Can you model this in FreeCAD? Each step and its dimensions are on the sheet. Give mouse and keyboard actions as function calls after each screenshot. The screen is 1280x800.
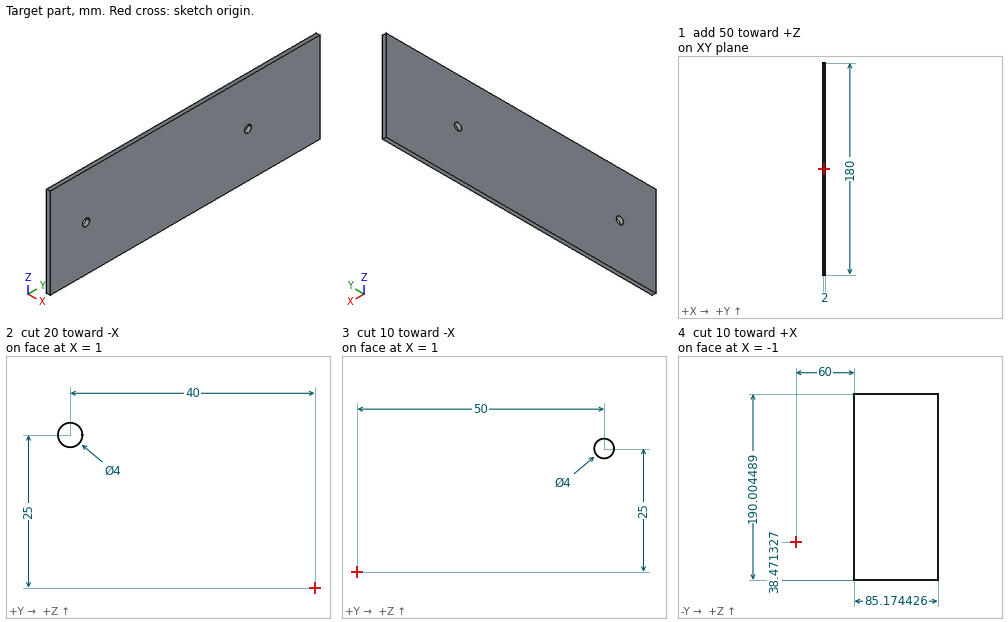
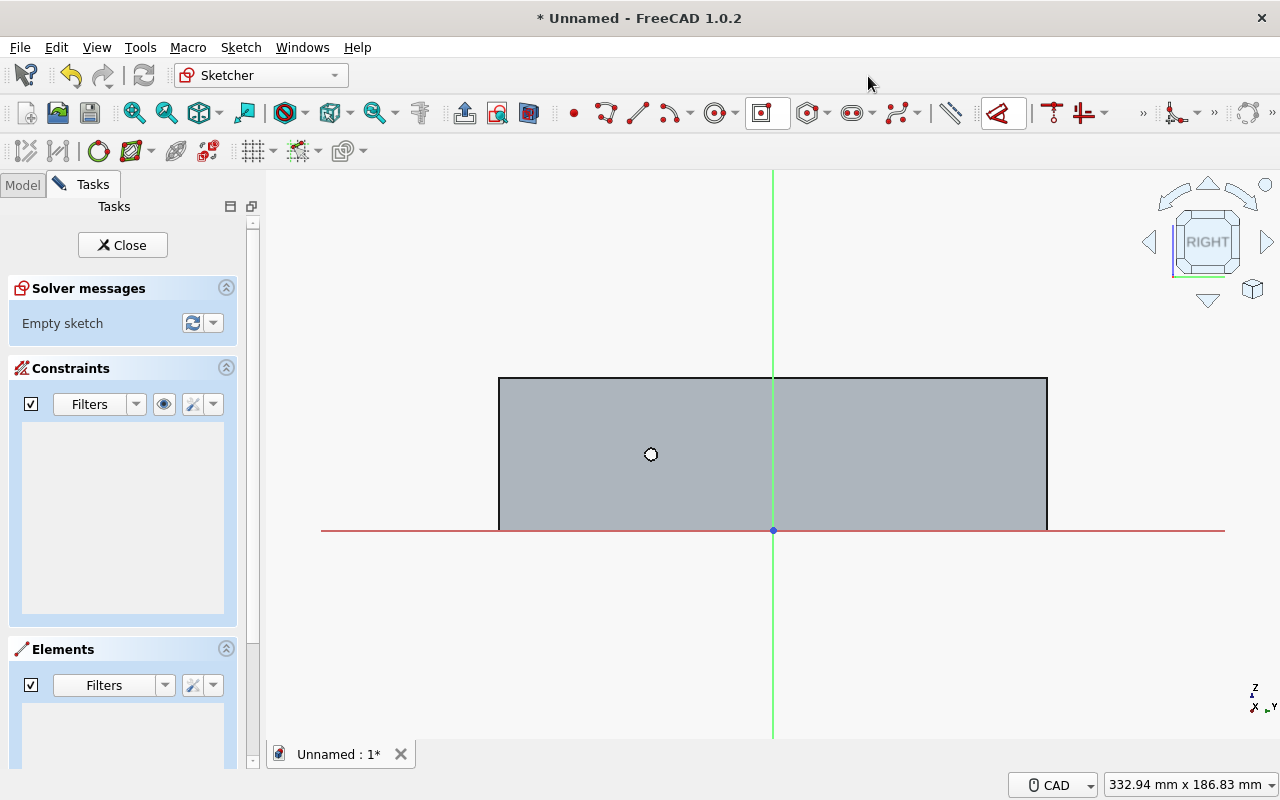
scroll(937, 455, up, 15)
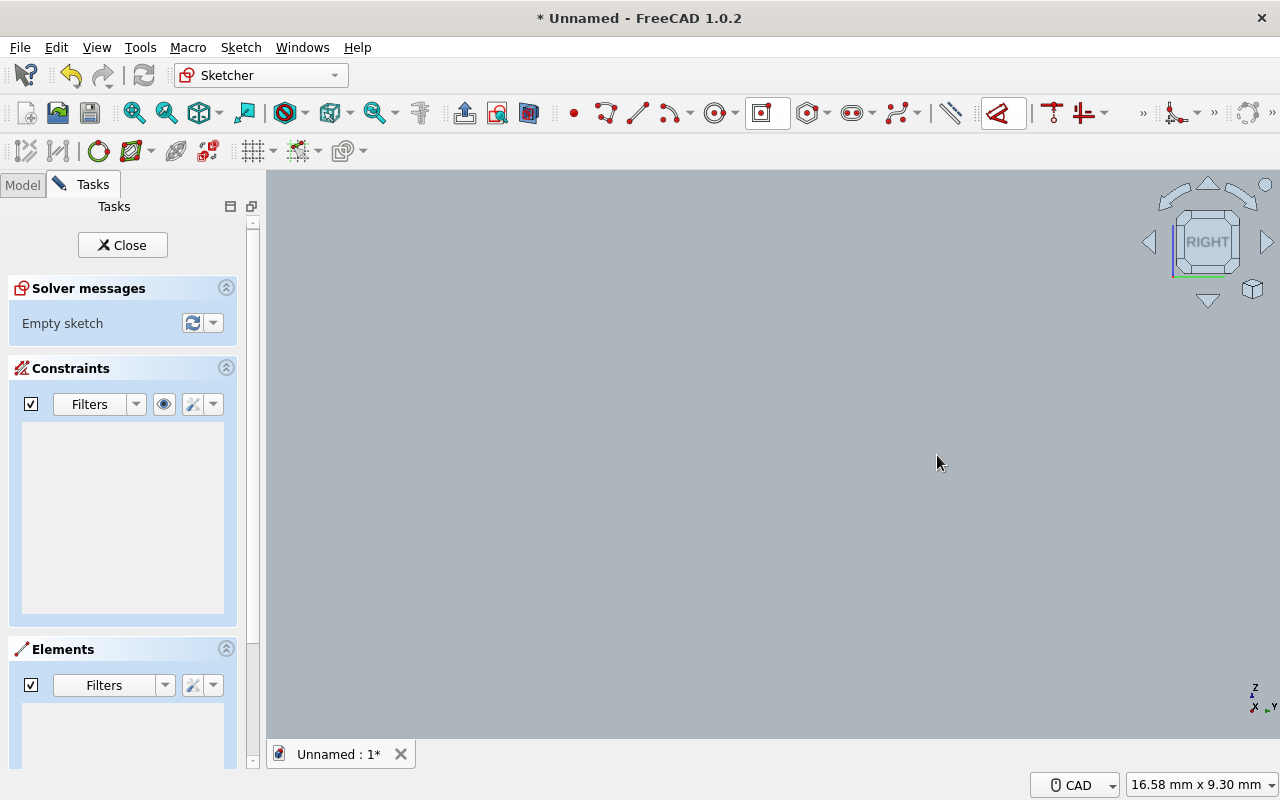
scroll(657, 397, up, 2)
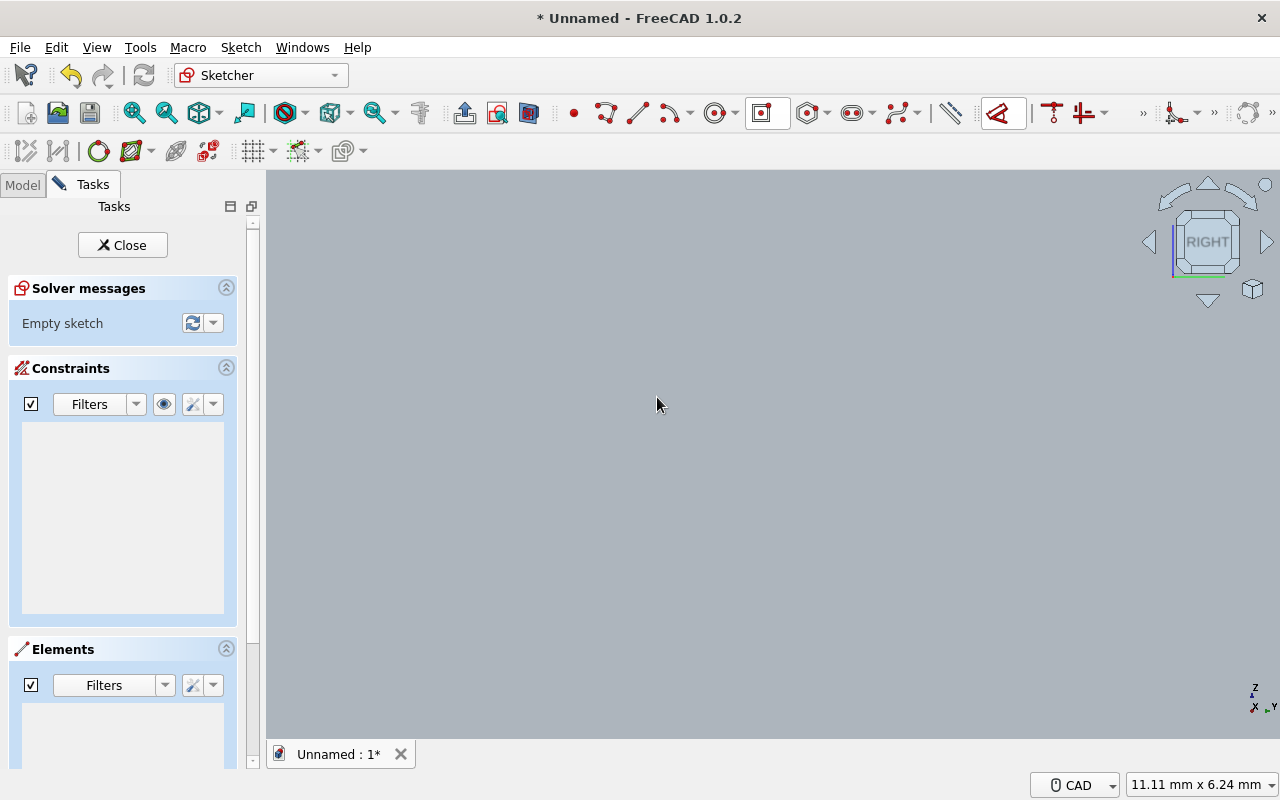
click(716, 114)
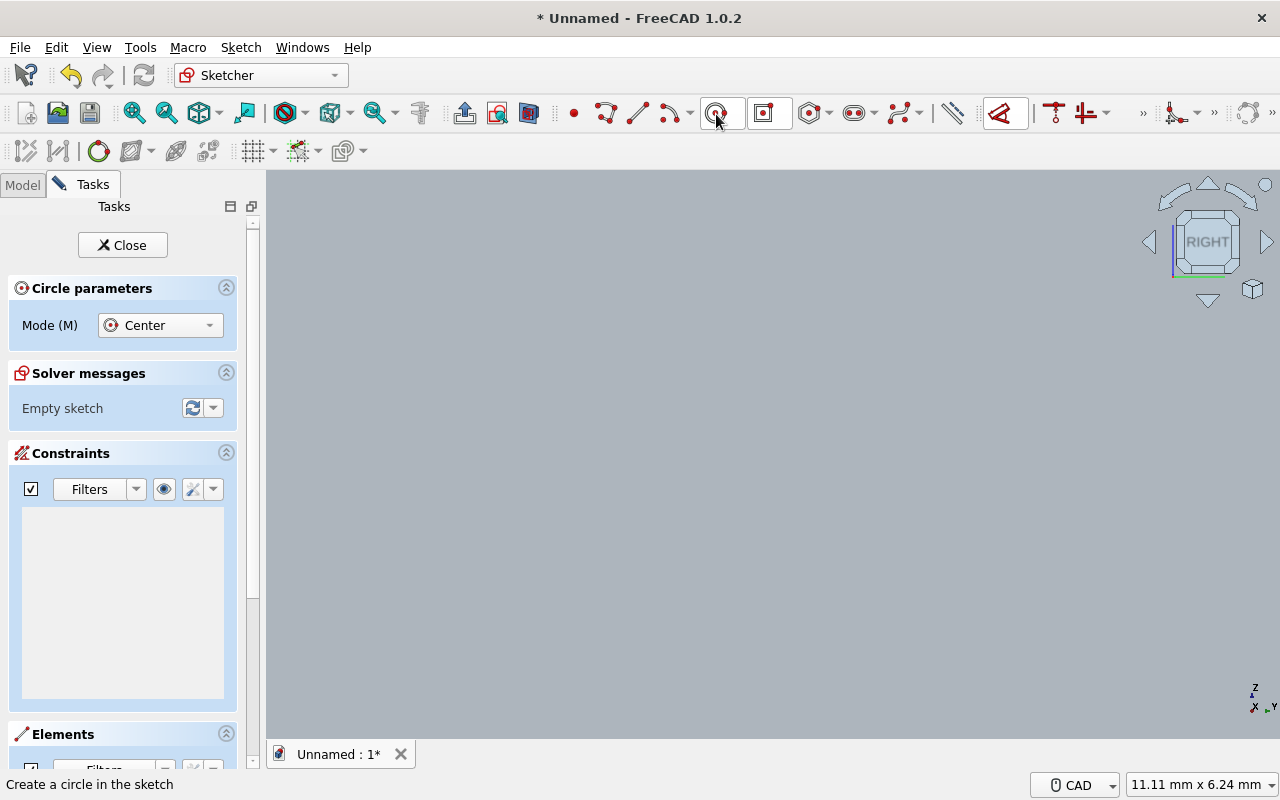
click(705, 454)
click(834, 325)
key(Escape)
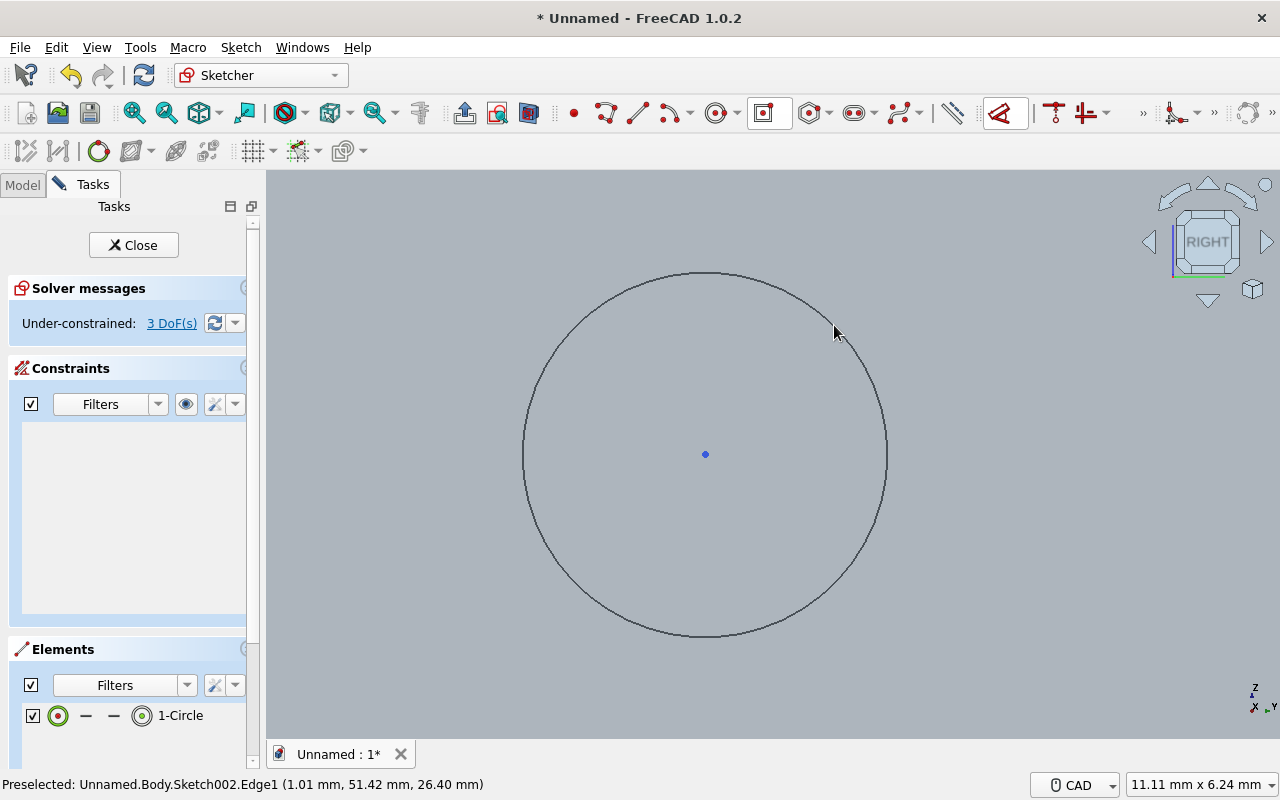
click(834, 326)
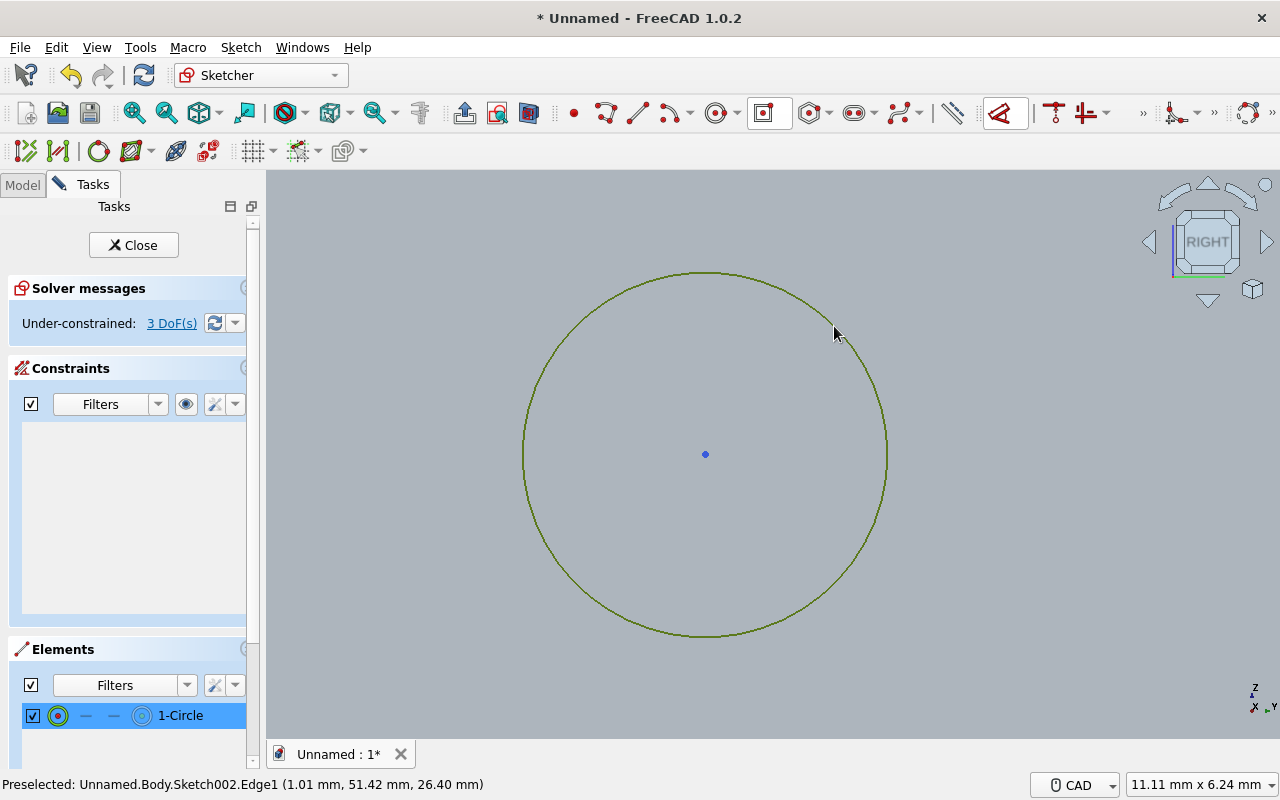
click(1022, 114)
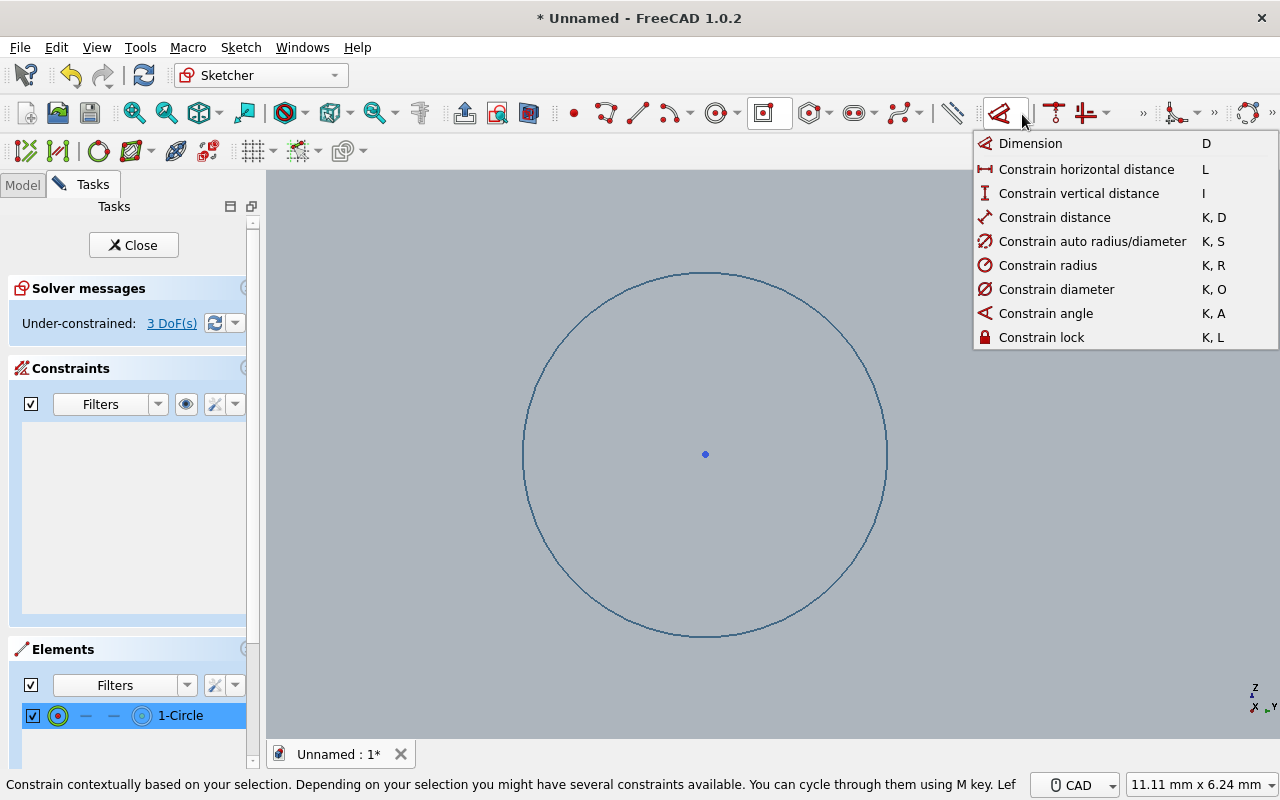
click(1126, 289)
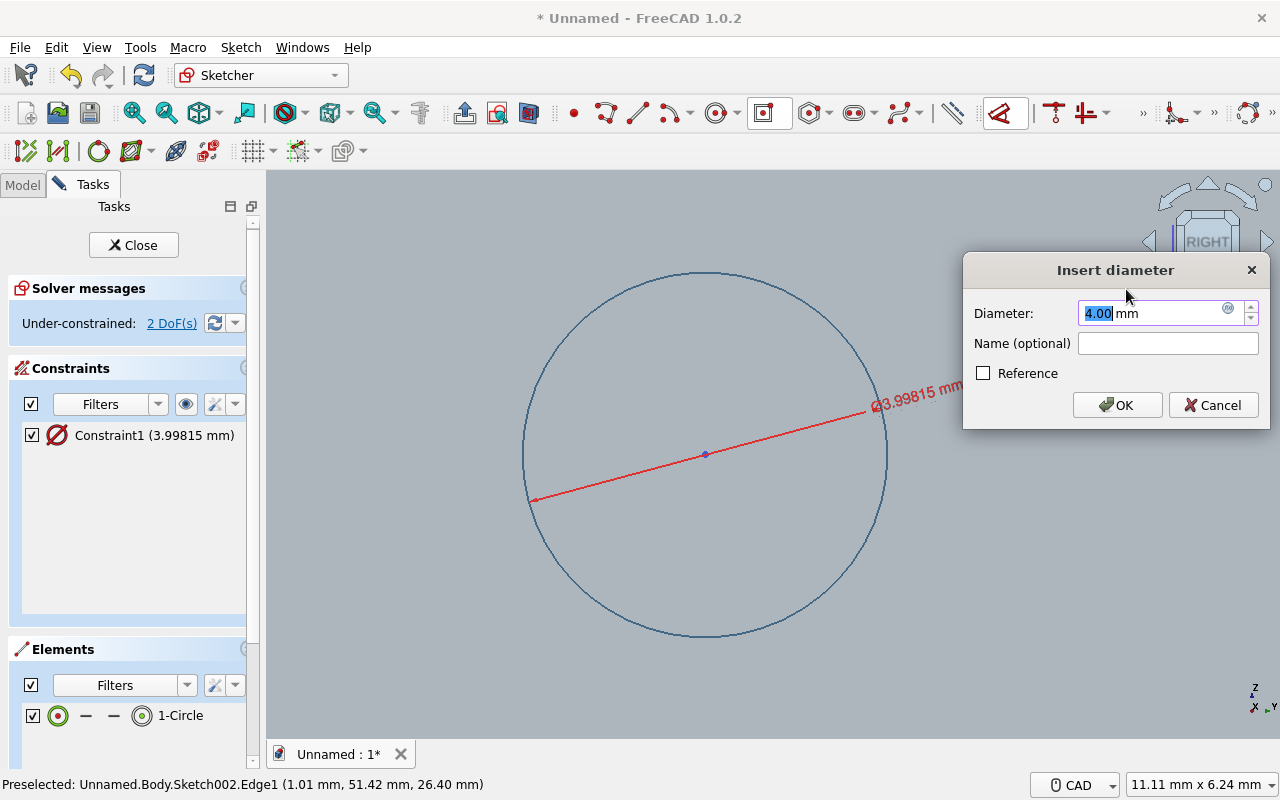
text(4)
key(Return)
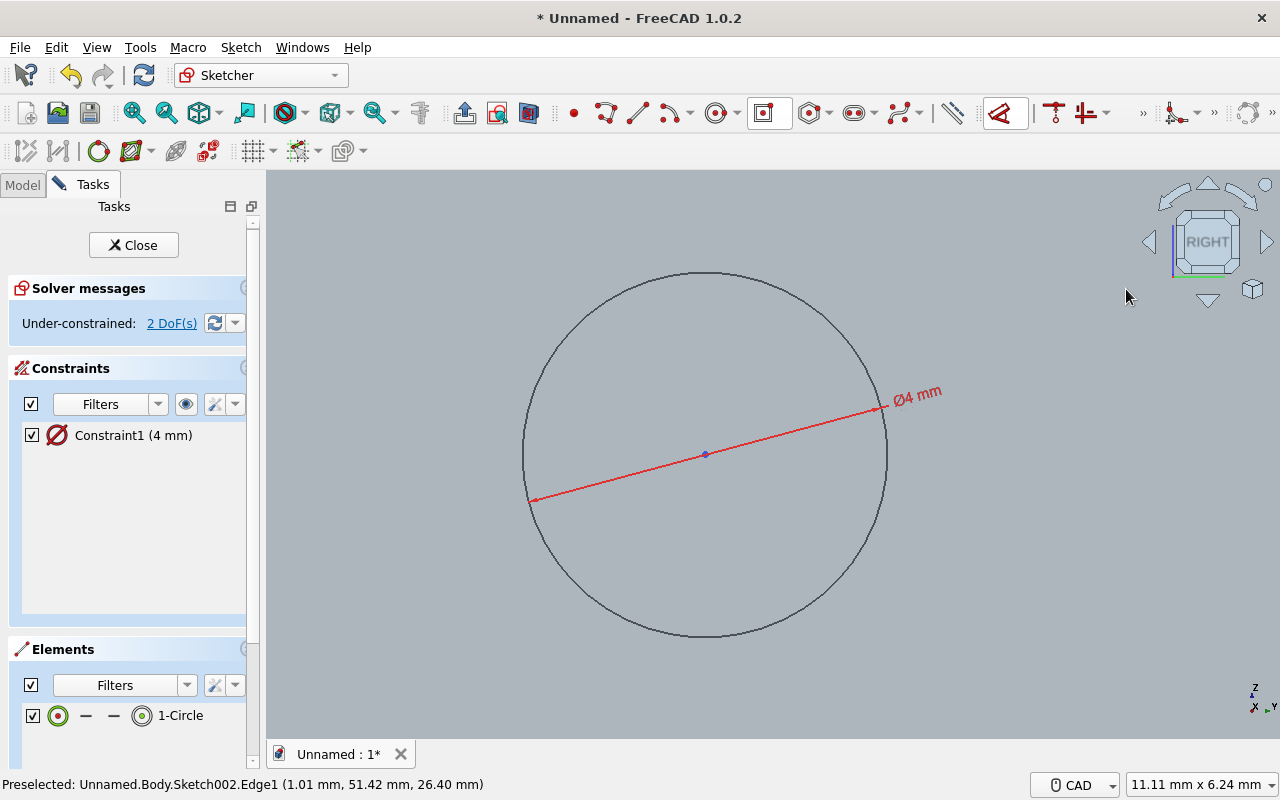
click(705, 455)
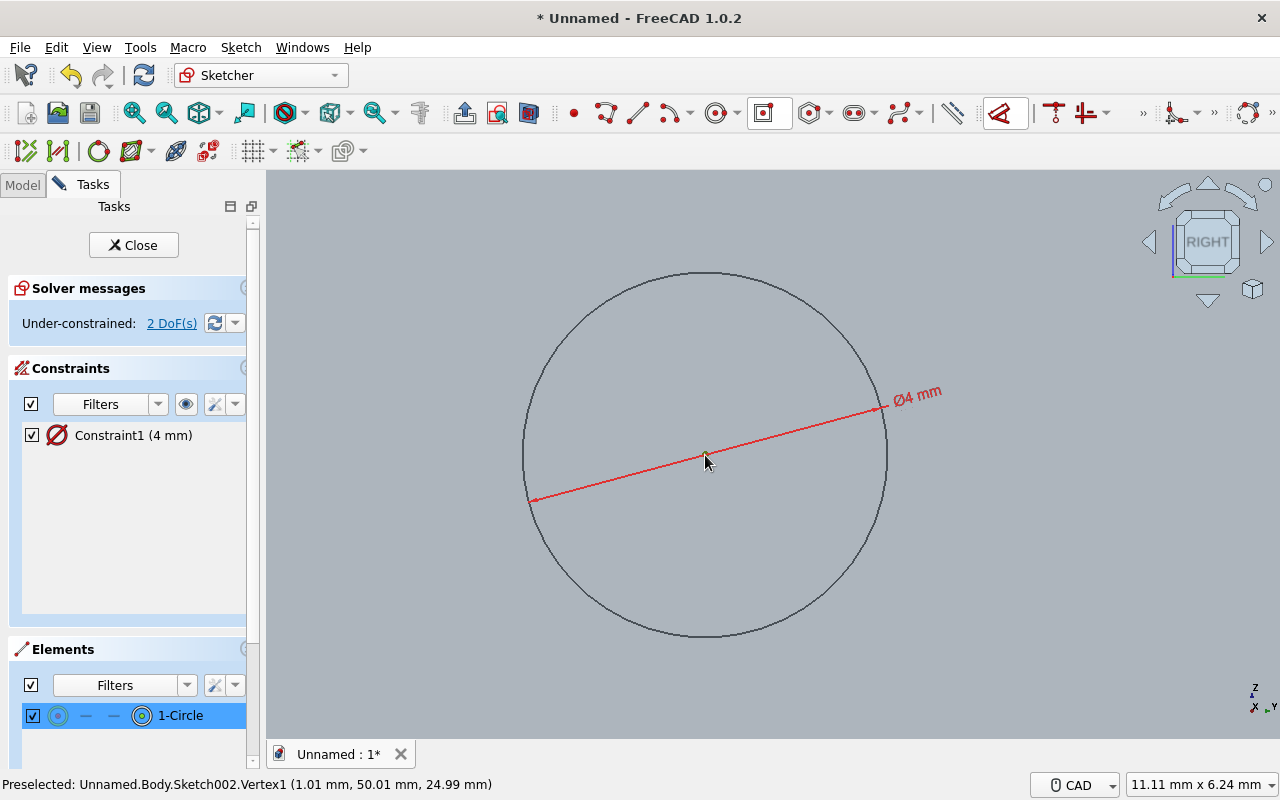
key(l)